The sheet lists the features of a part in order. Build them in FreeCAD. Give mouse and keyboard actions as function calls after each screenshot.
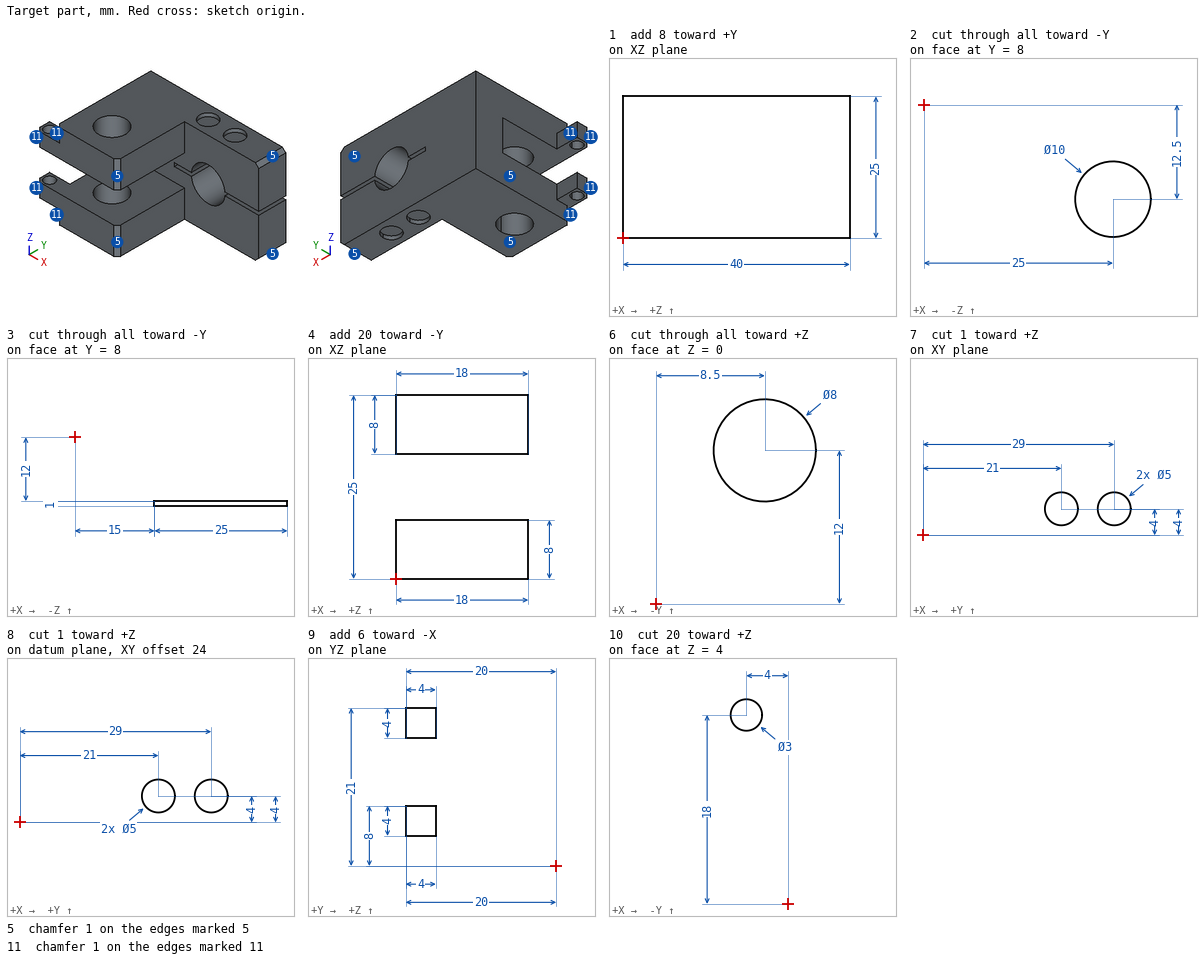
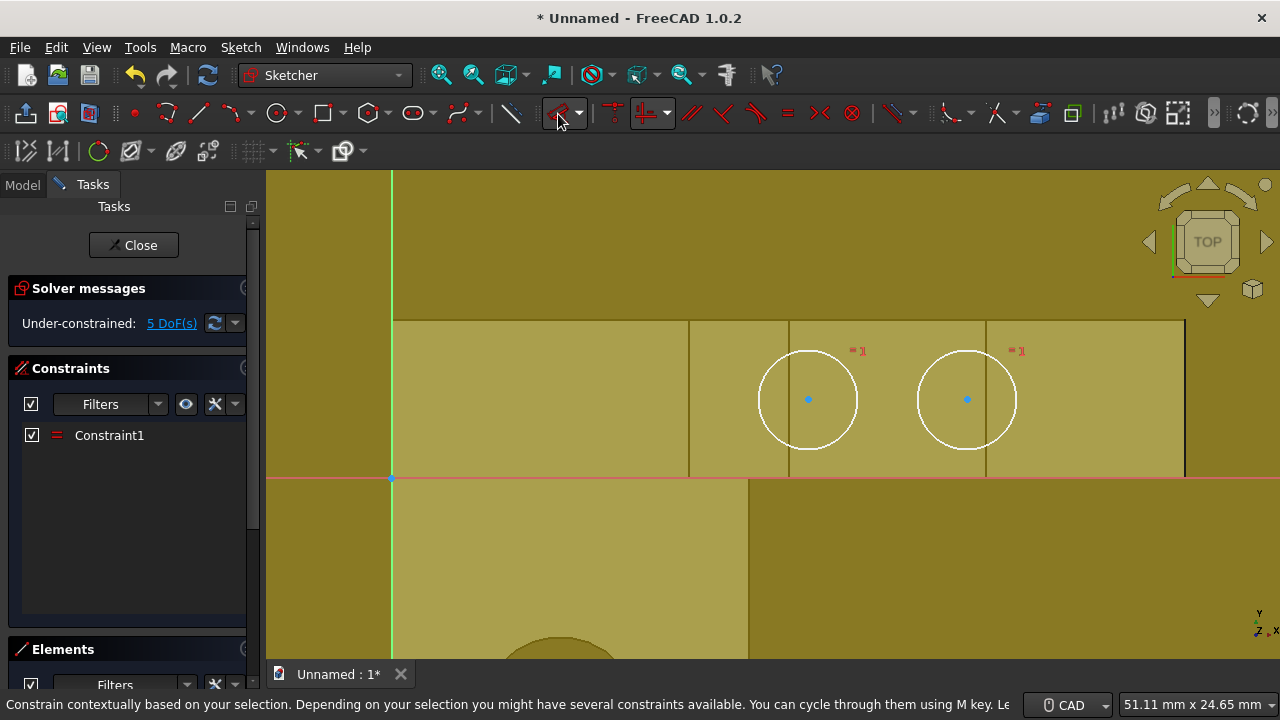
click(843, 365)
click(866, 342)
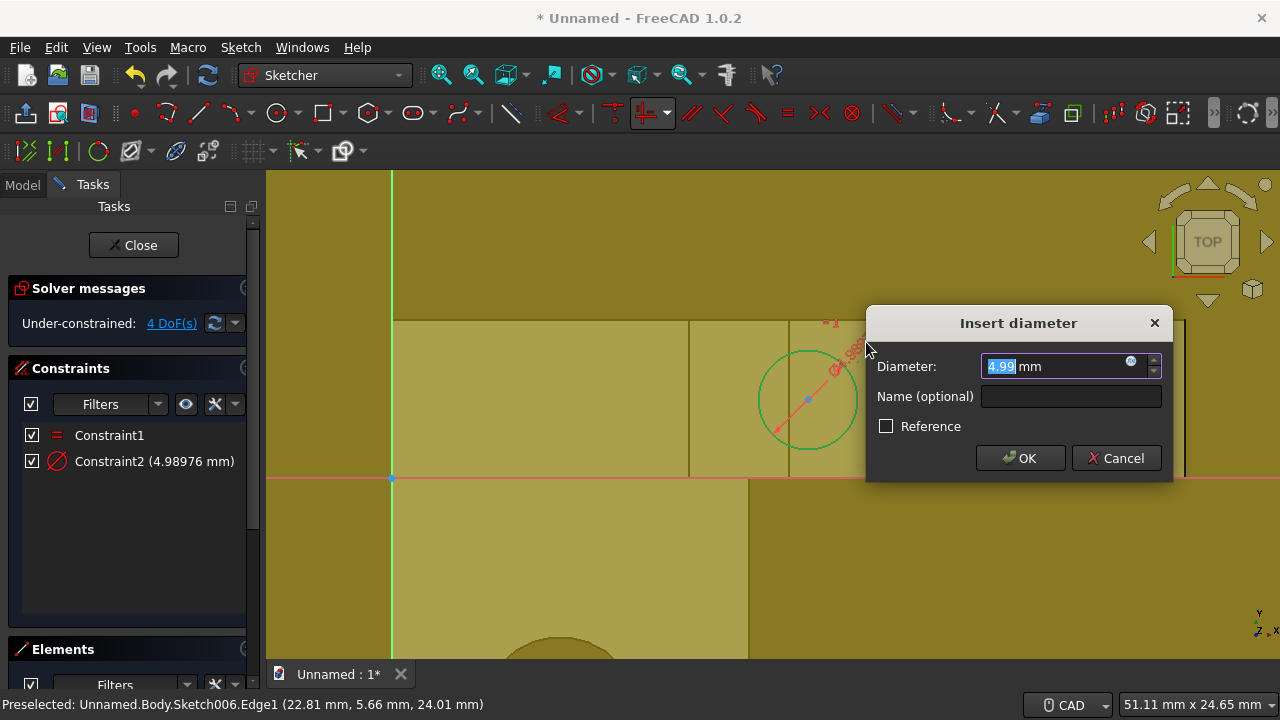
text(5)
key(Return)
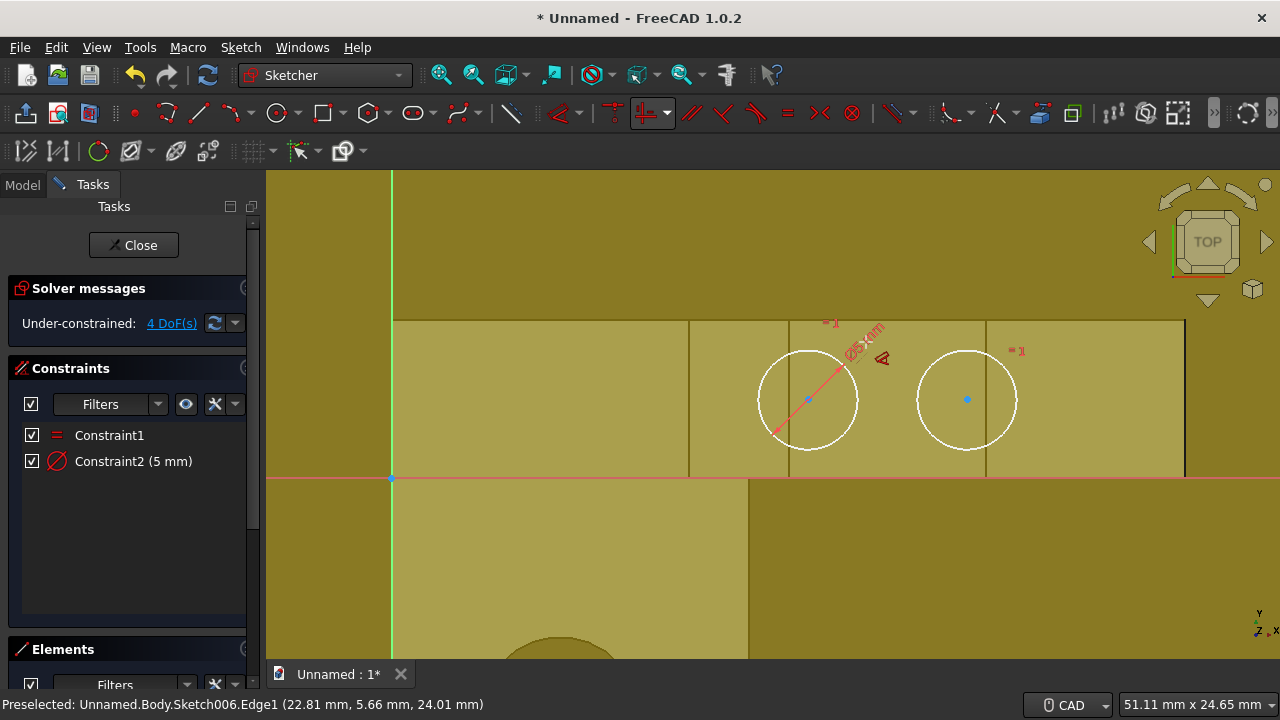
click(808, 400)
click(358, 439)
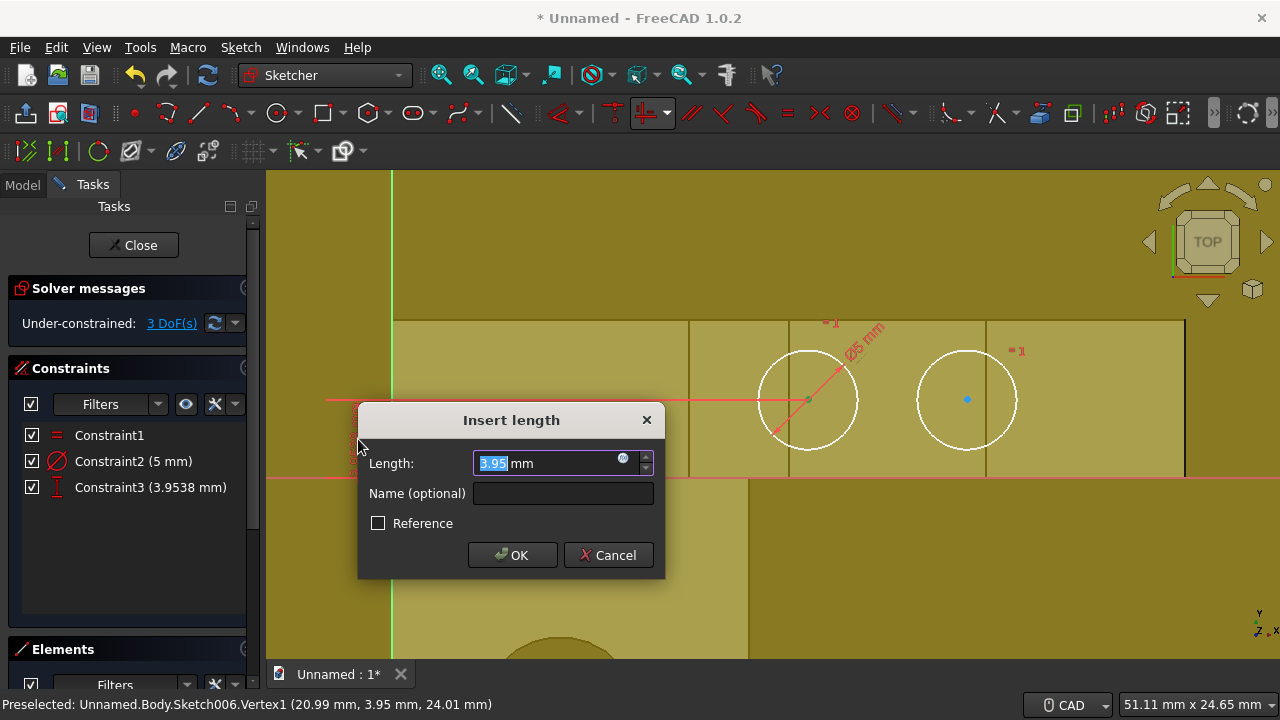
text(4)
key(Return)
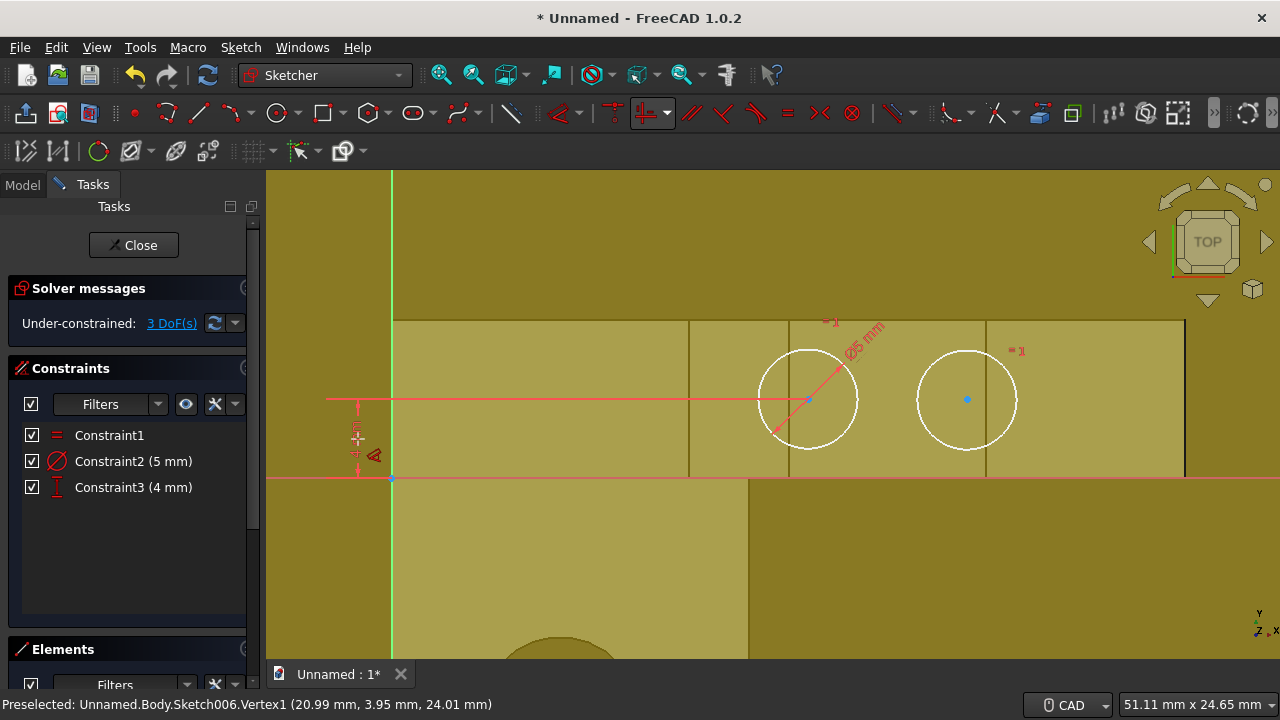
click(967, 400)
click(358, 412)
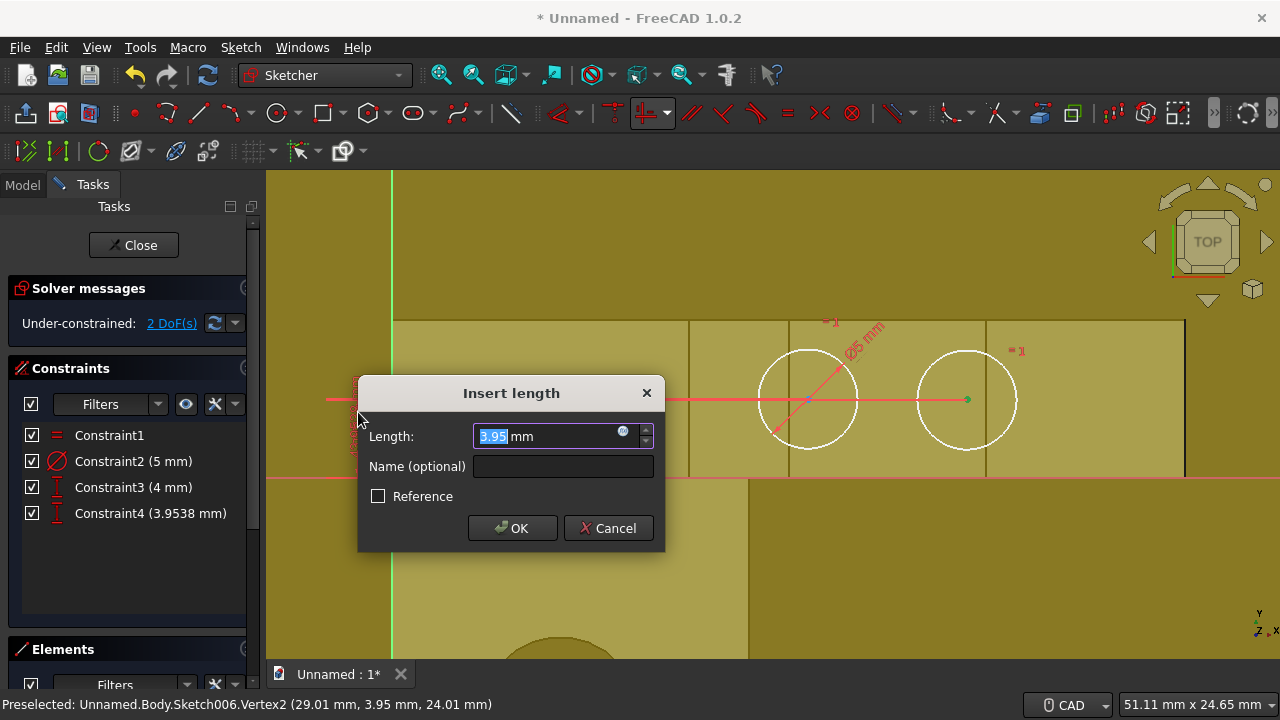
text(4)
key(Return)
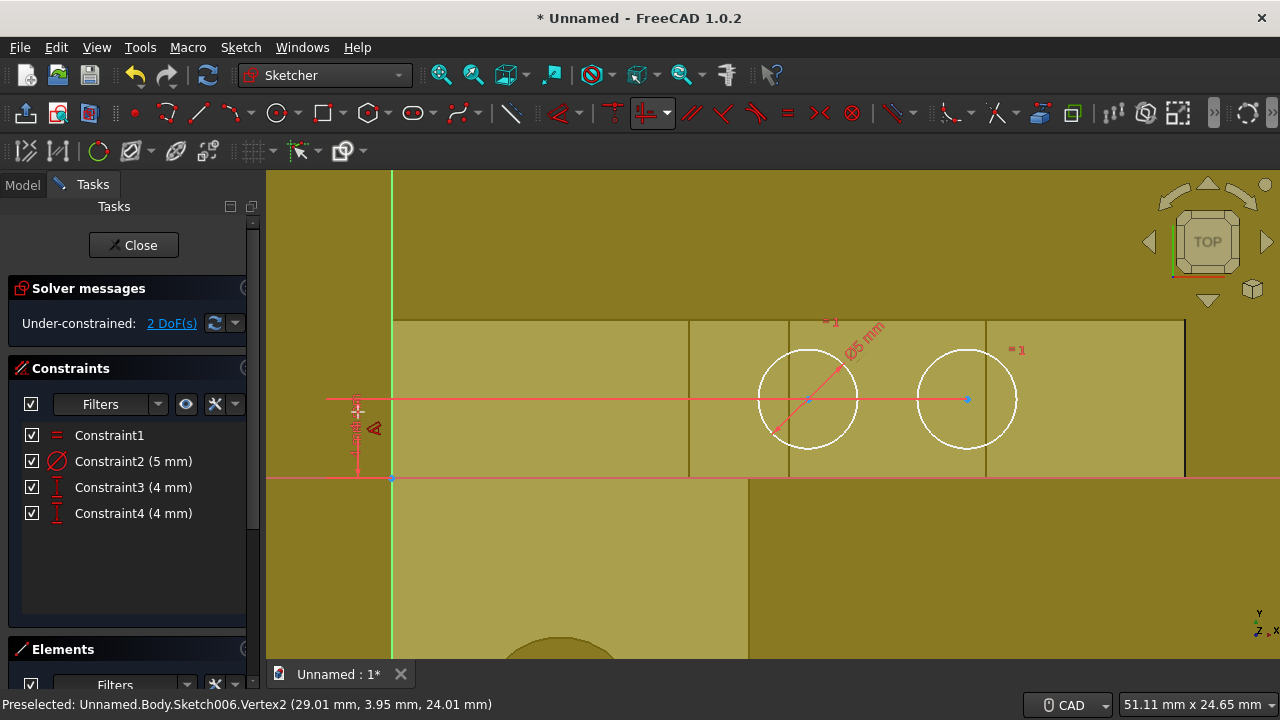
click(808, 399)
click(600, 512)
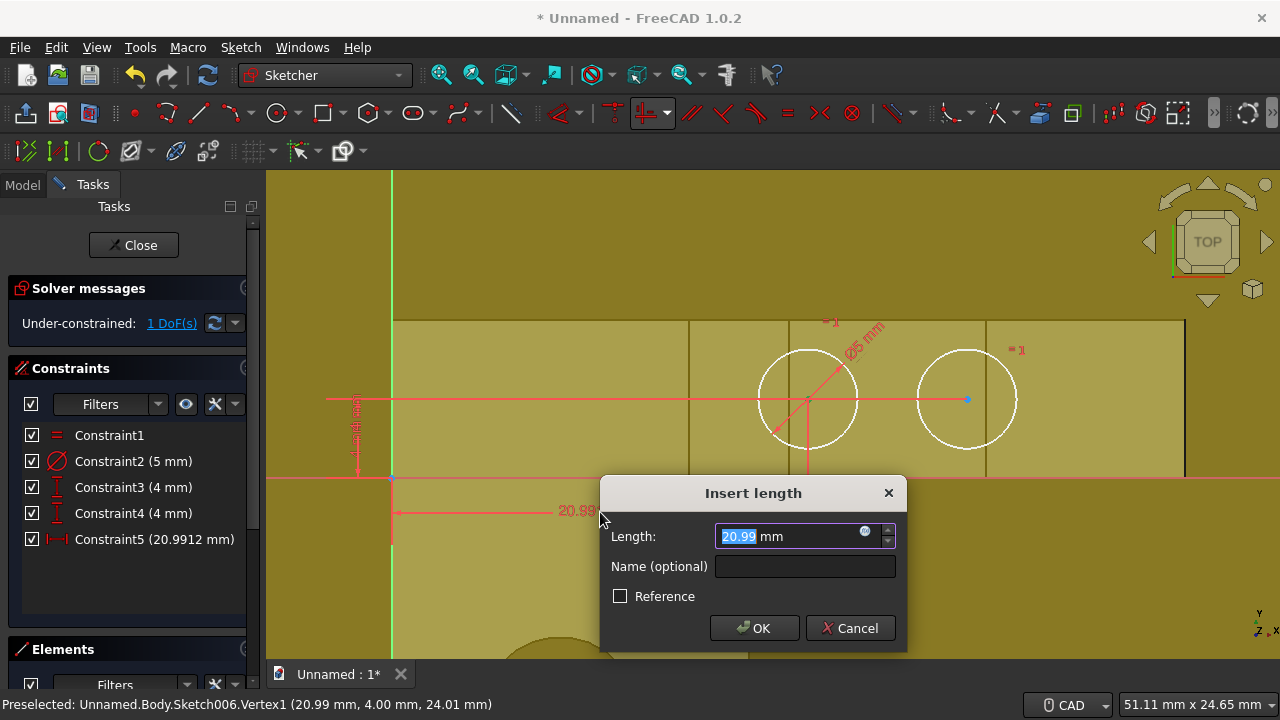
text(21)
key(Return)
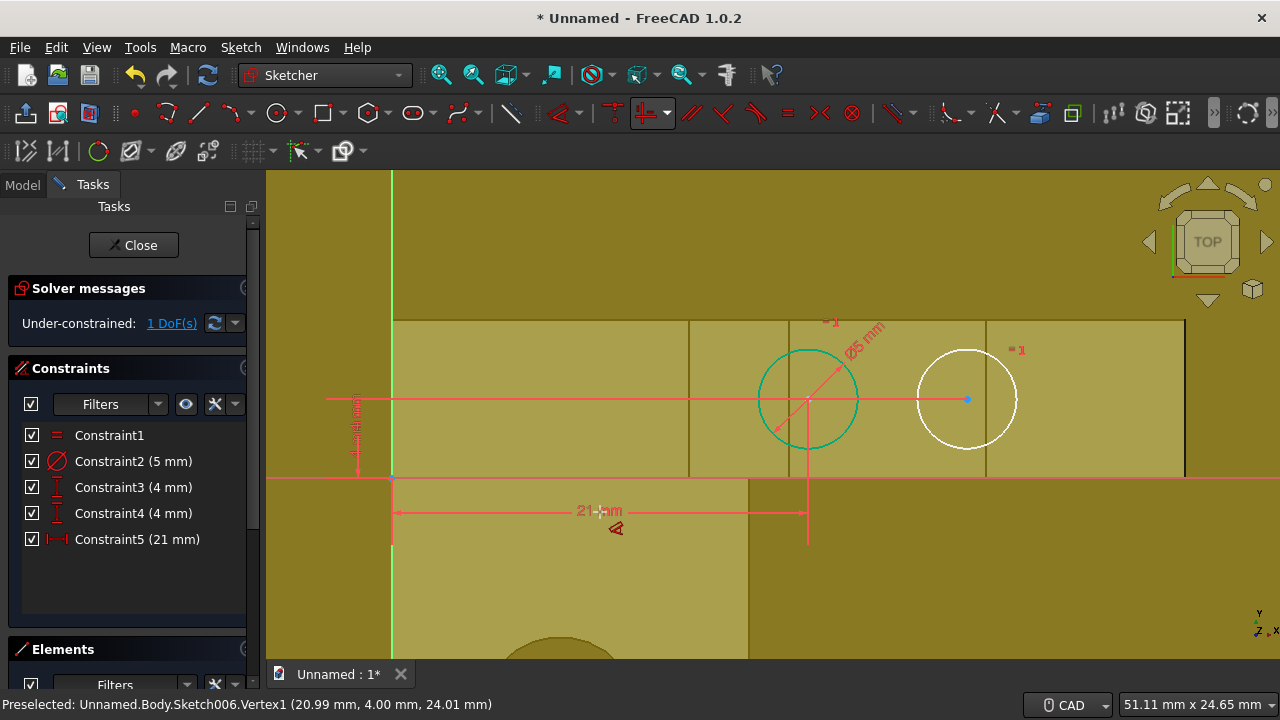
click(967, 399)
click(679, 512)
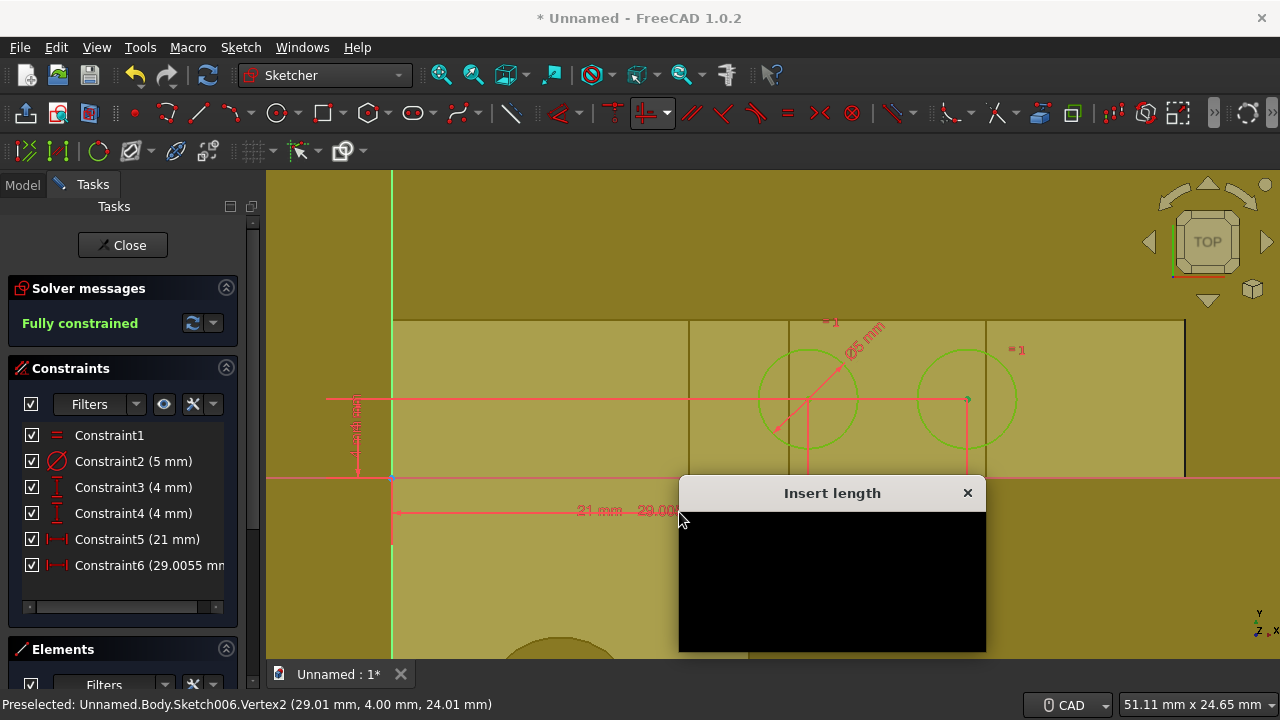
text(29)
key(Return)
key(Escape)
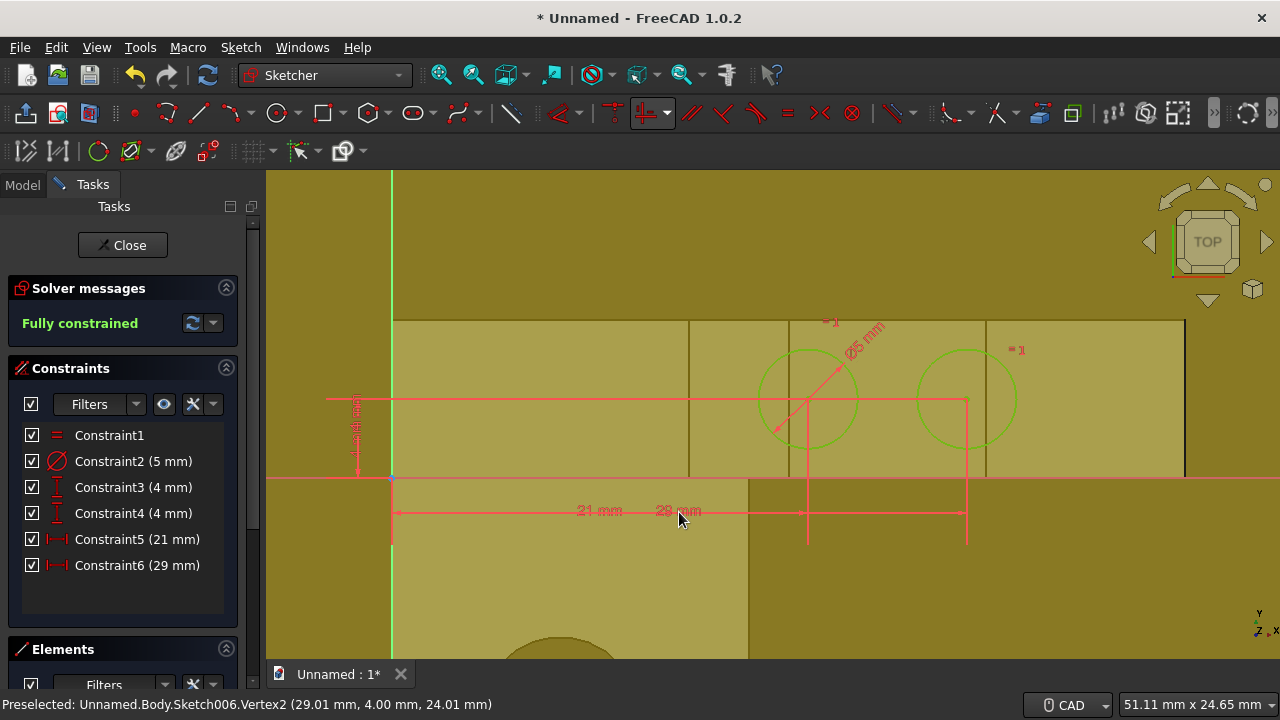
click(123, 245)